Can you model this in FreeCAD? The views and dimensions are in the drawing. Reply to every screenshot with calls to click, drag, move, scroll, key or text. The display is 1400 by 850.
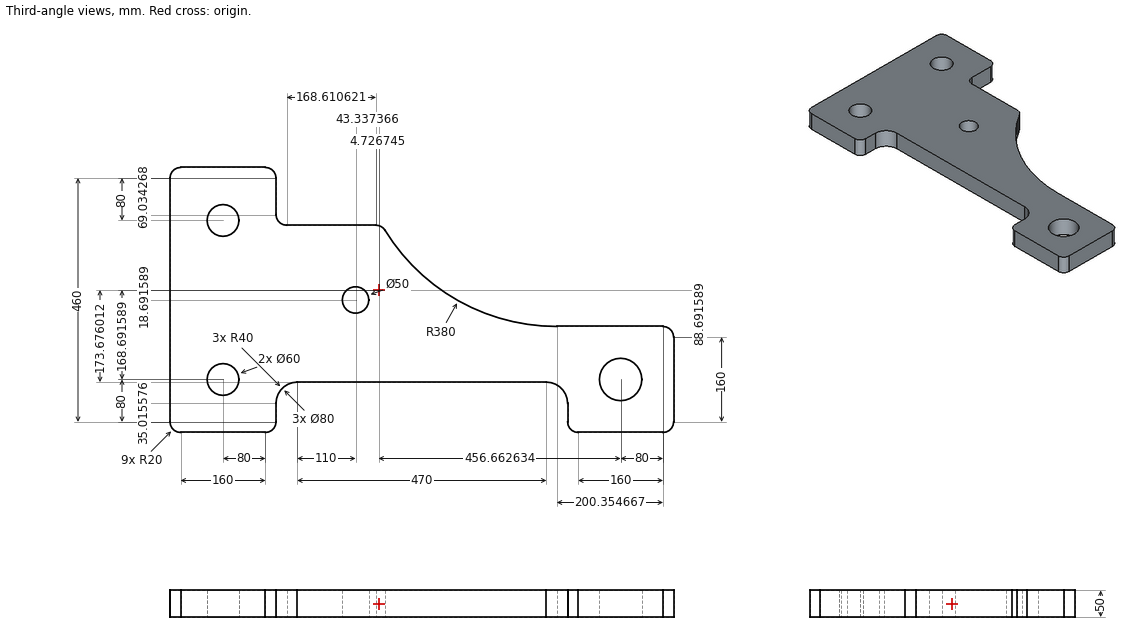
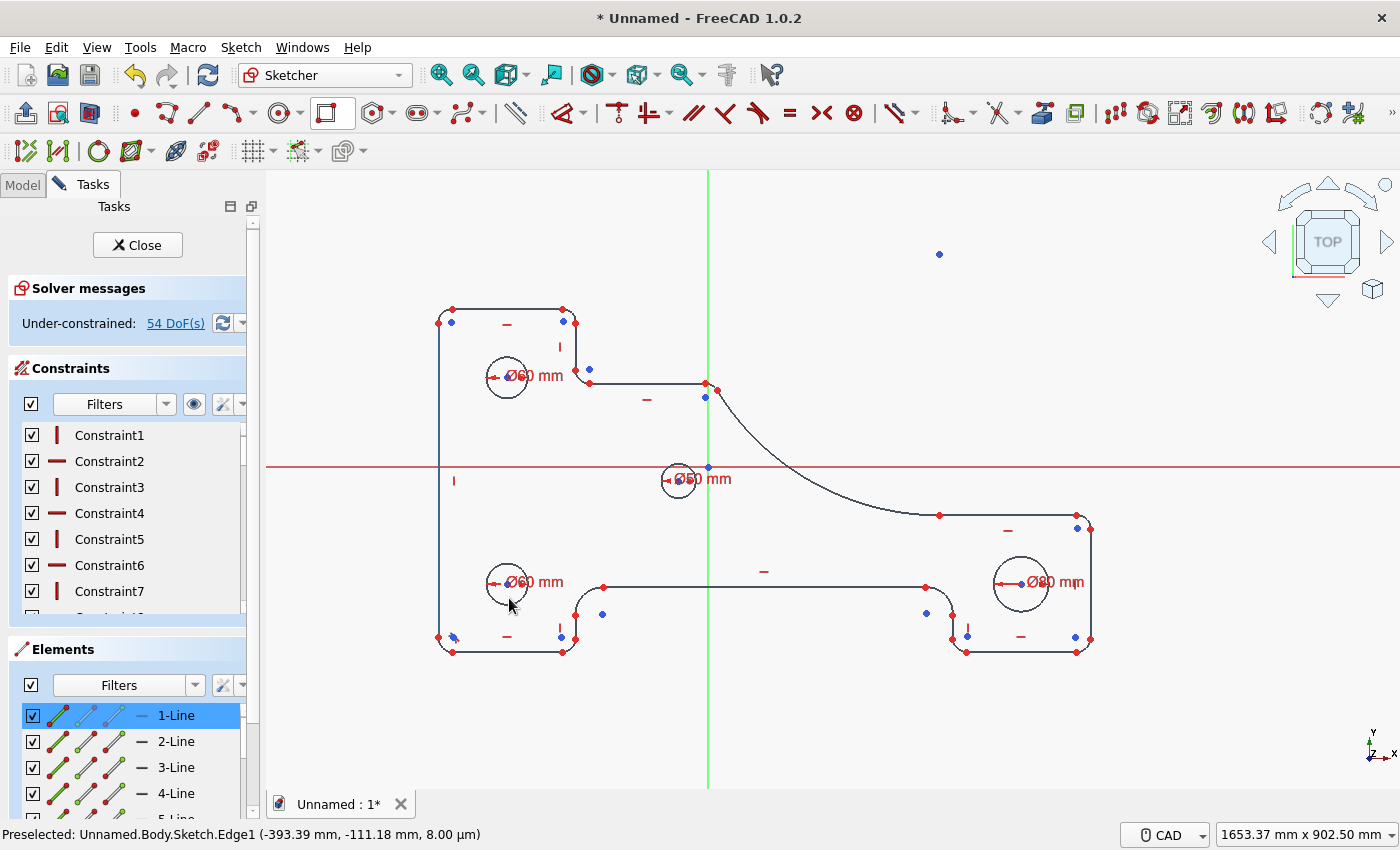
scroll(446, 311, up, 4)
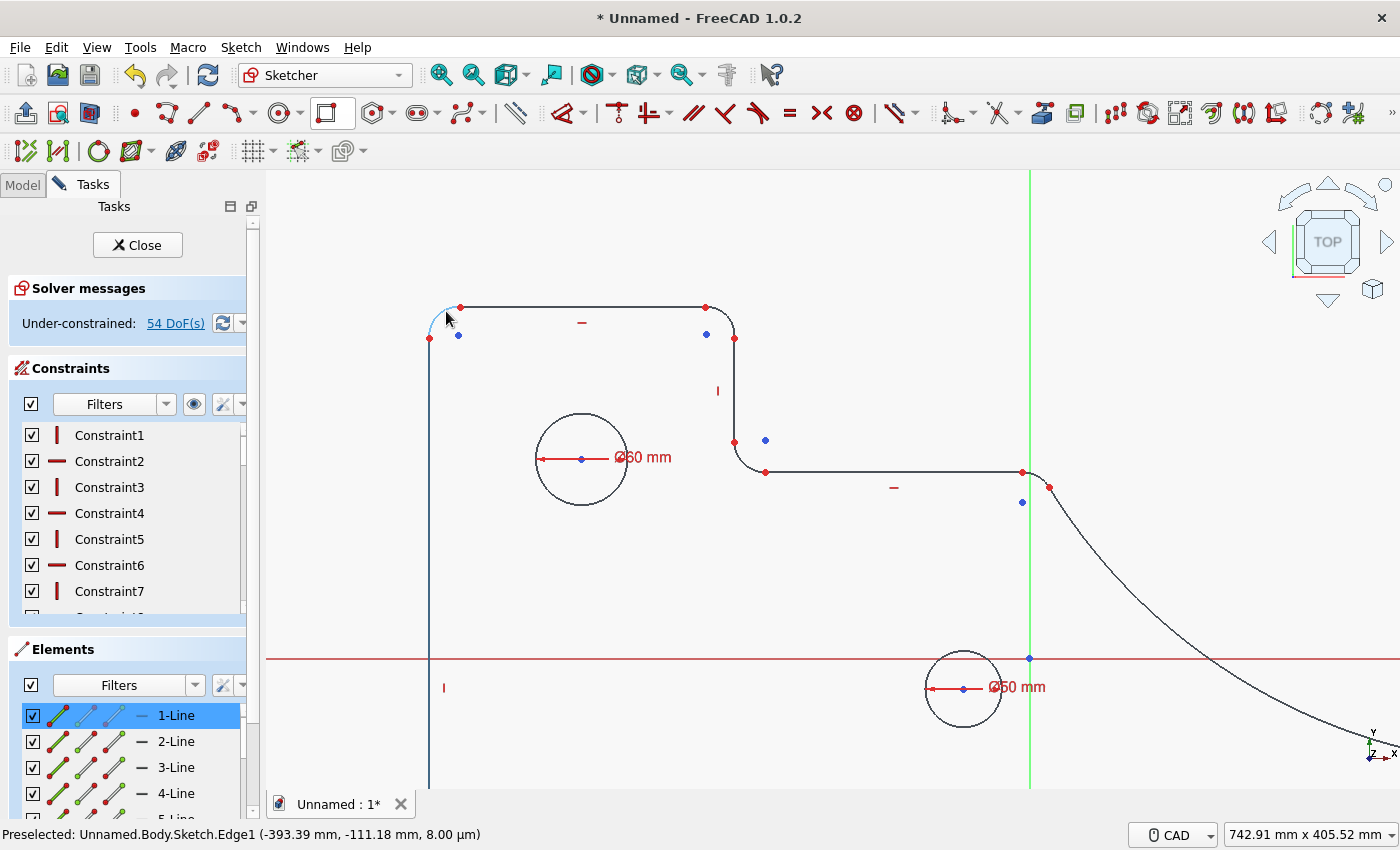
click(446, 310)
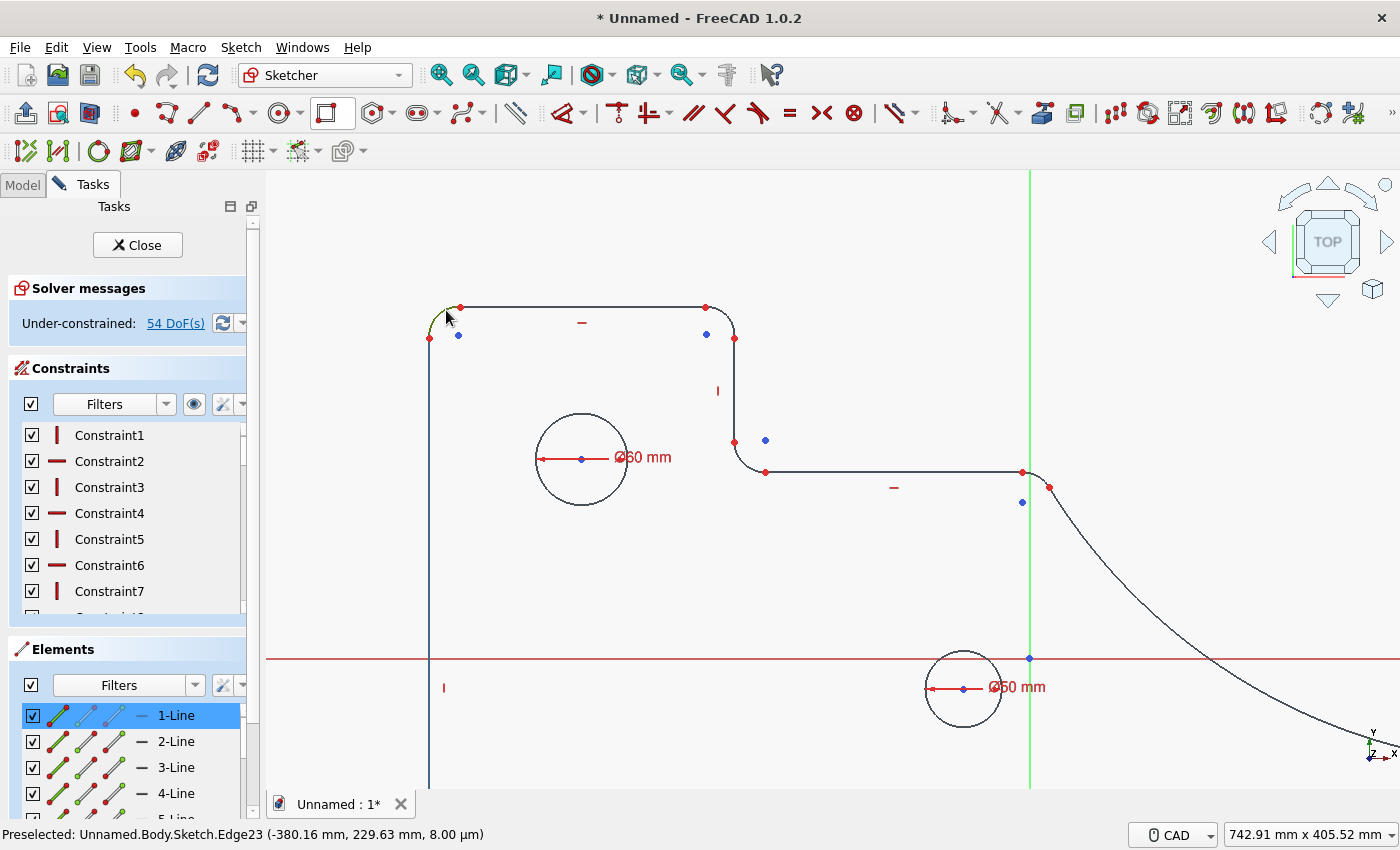
click(758, 114)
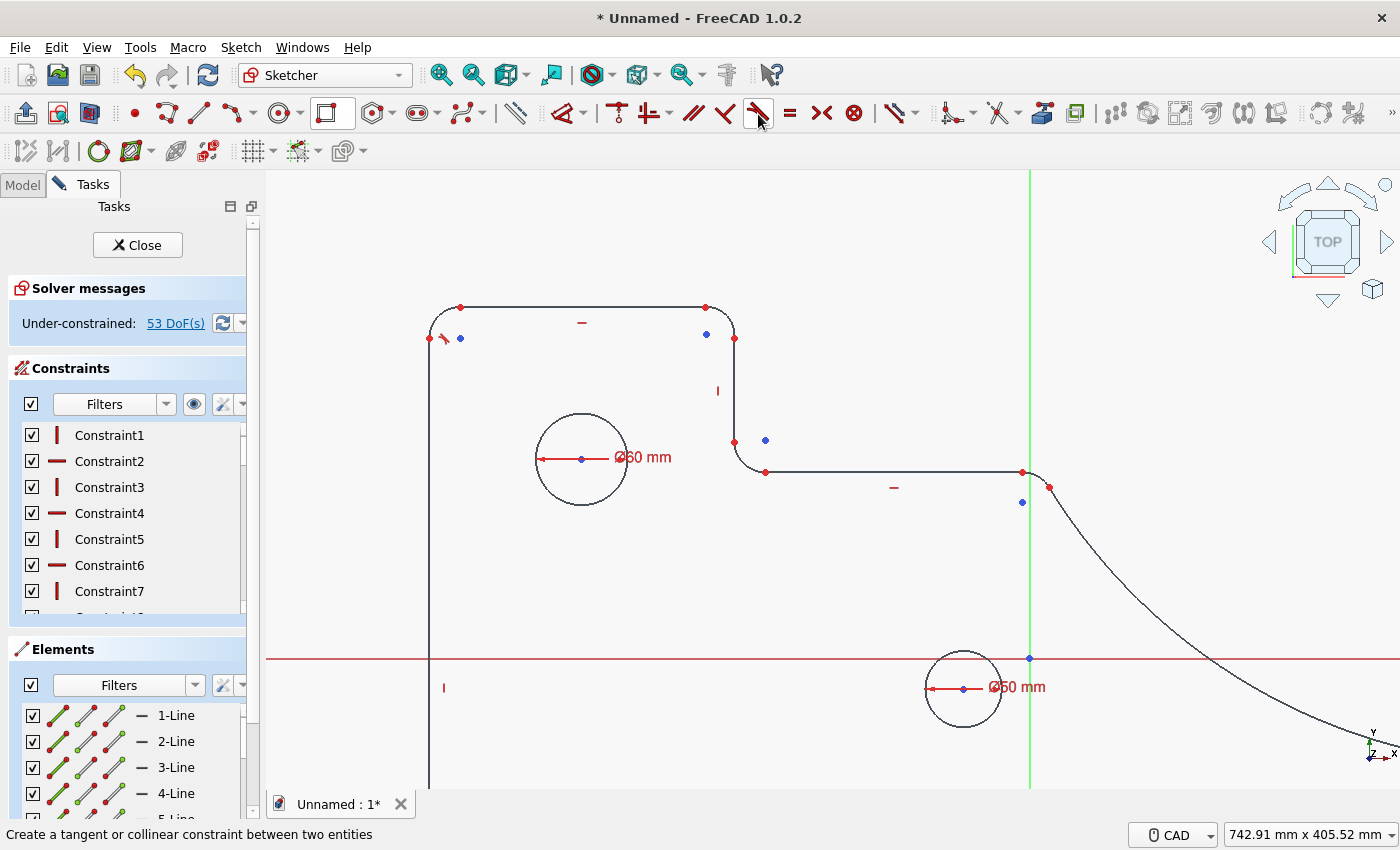
scroll(446, 310, down, 4)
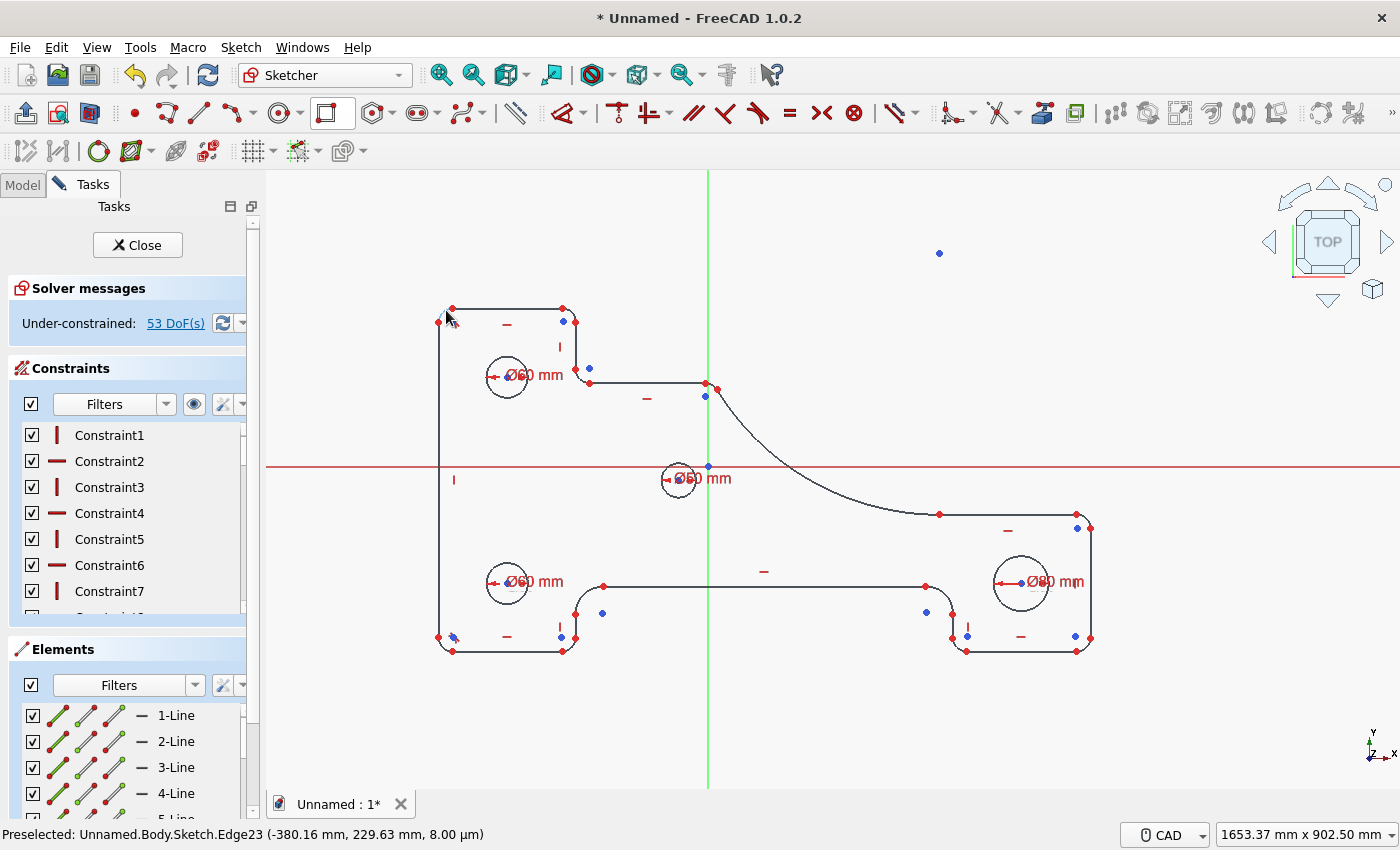
click(486, 652)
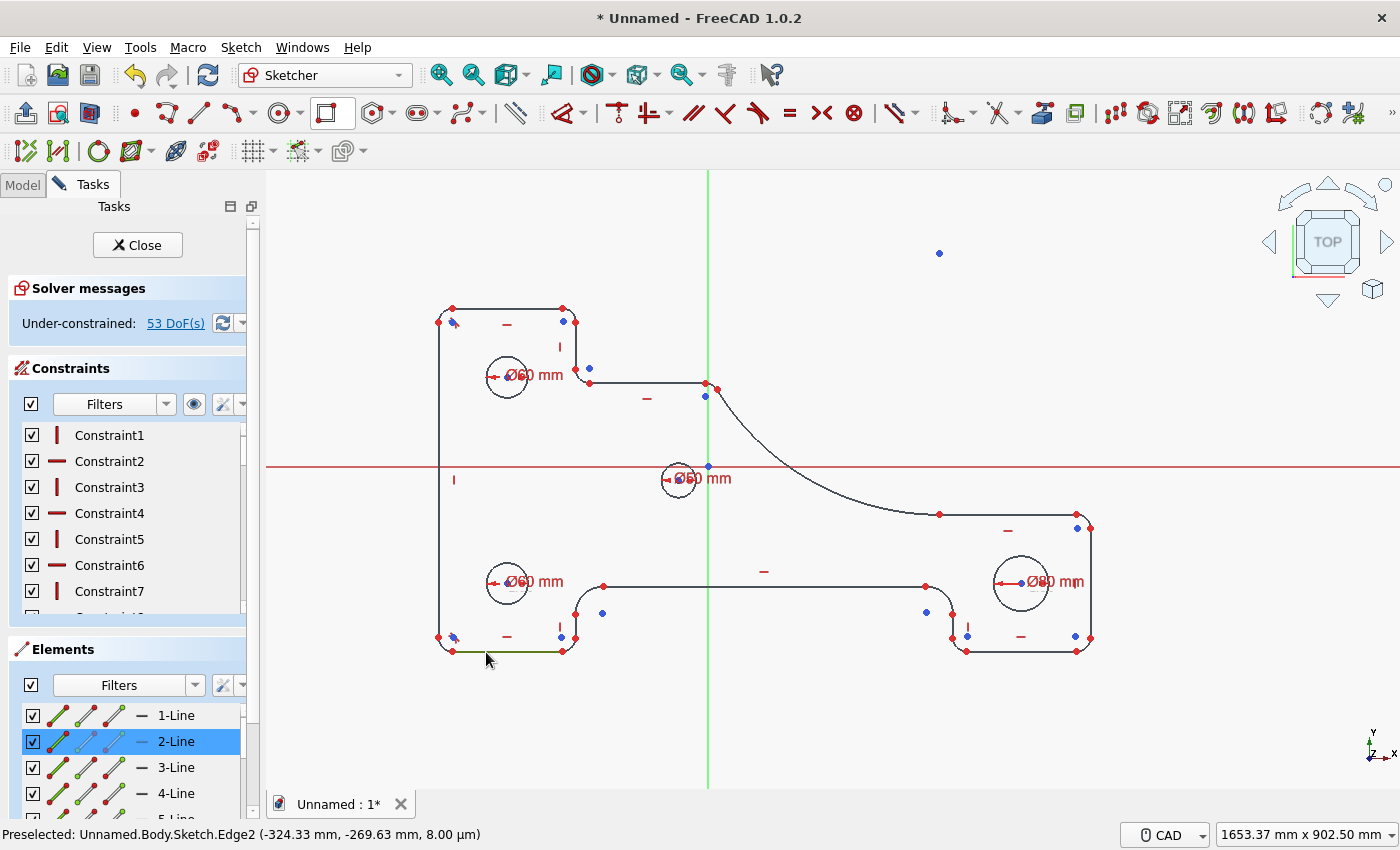
scroll(443, 647, up, 2)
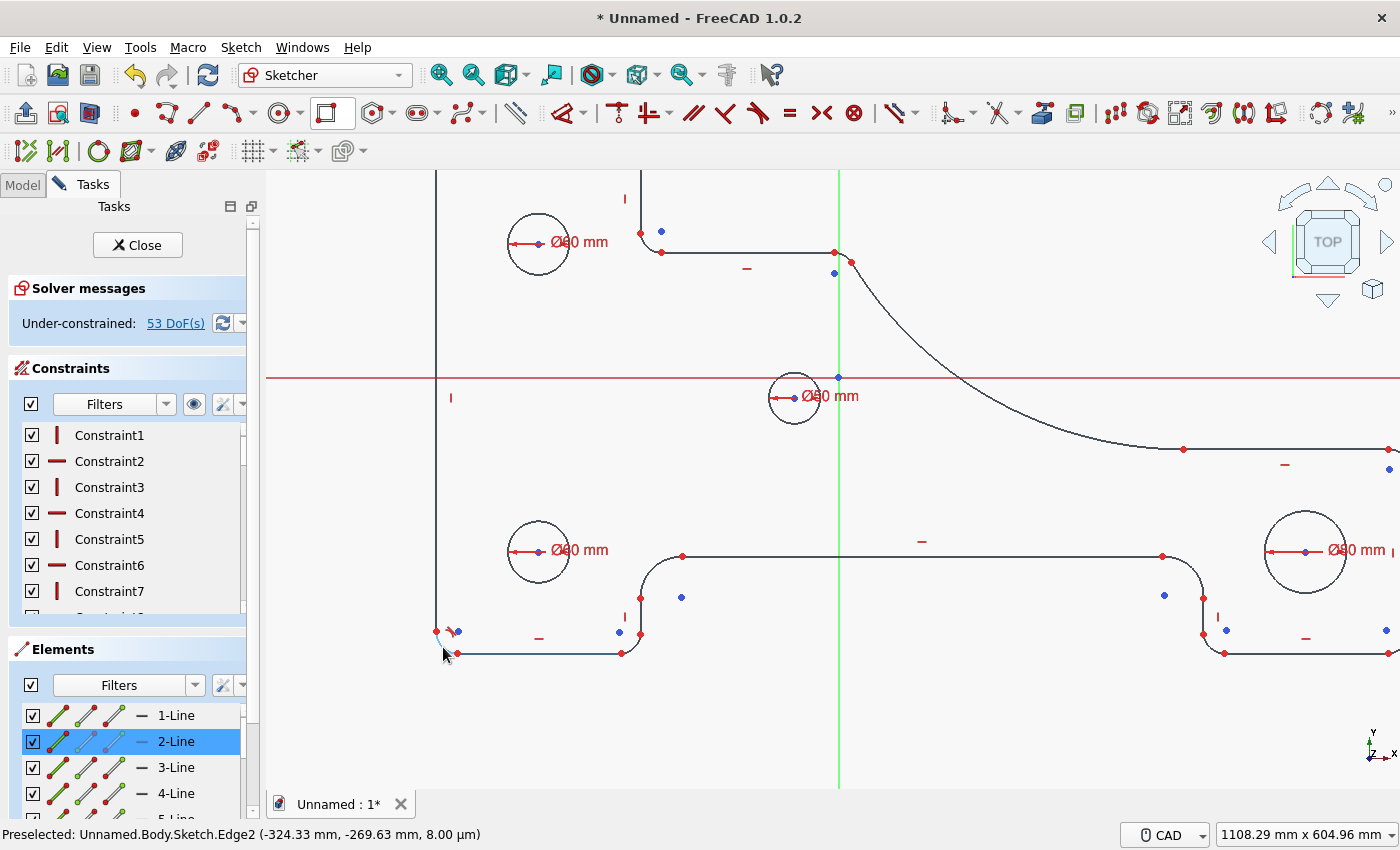
click(442, 647)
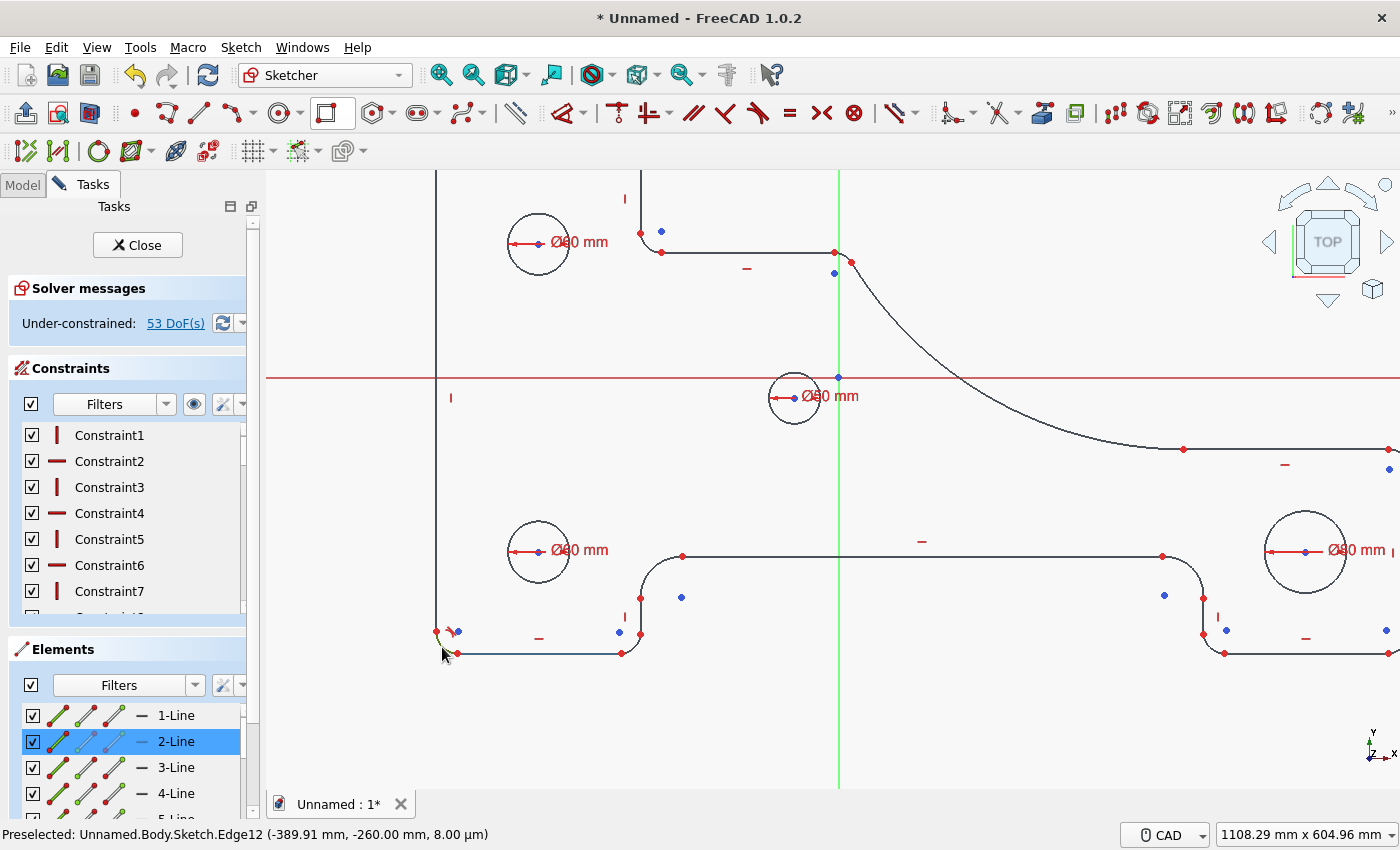
click(758, 114)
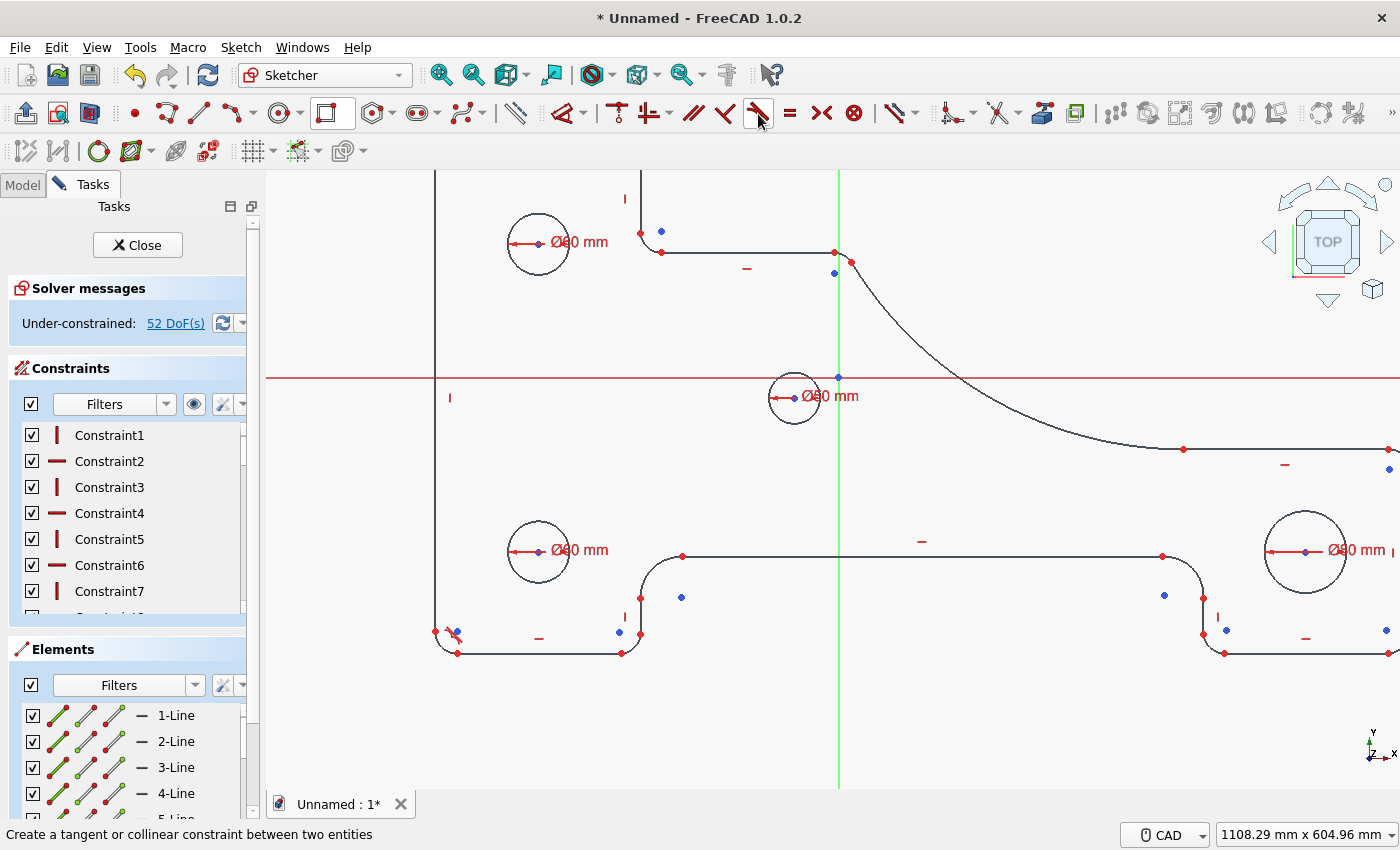
click(506, 654)